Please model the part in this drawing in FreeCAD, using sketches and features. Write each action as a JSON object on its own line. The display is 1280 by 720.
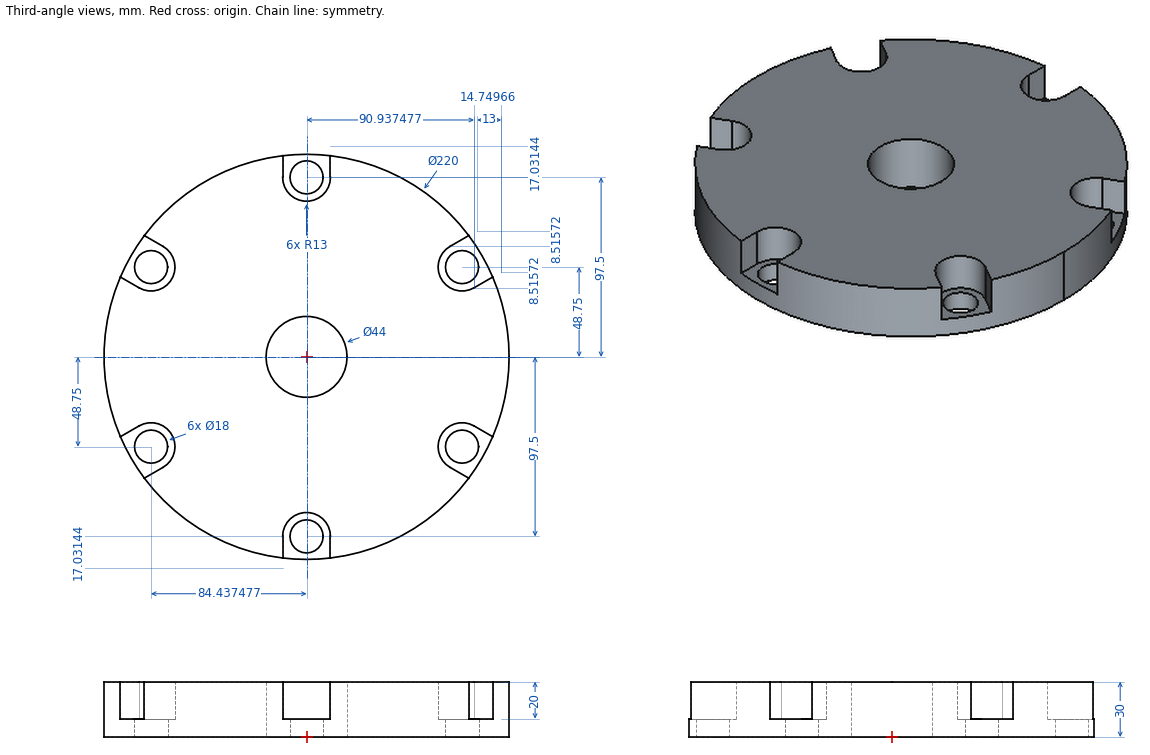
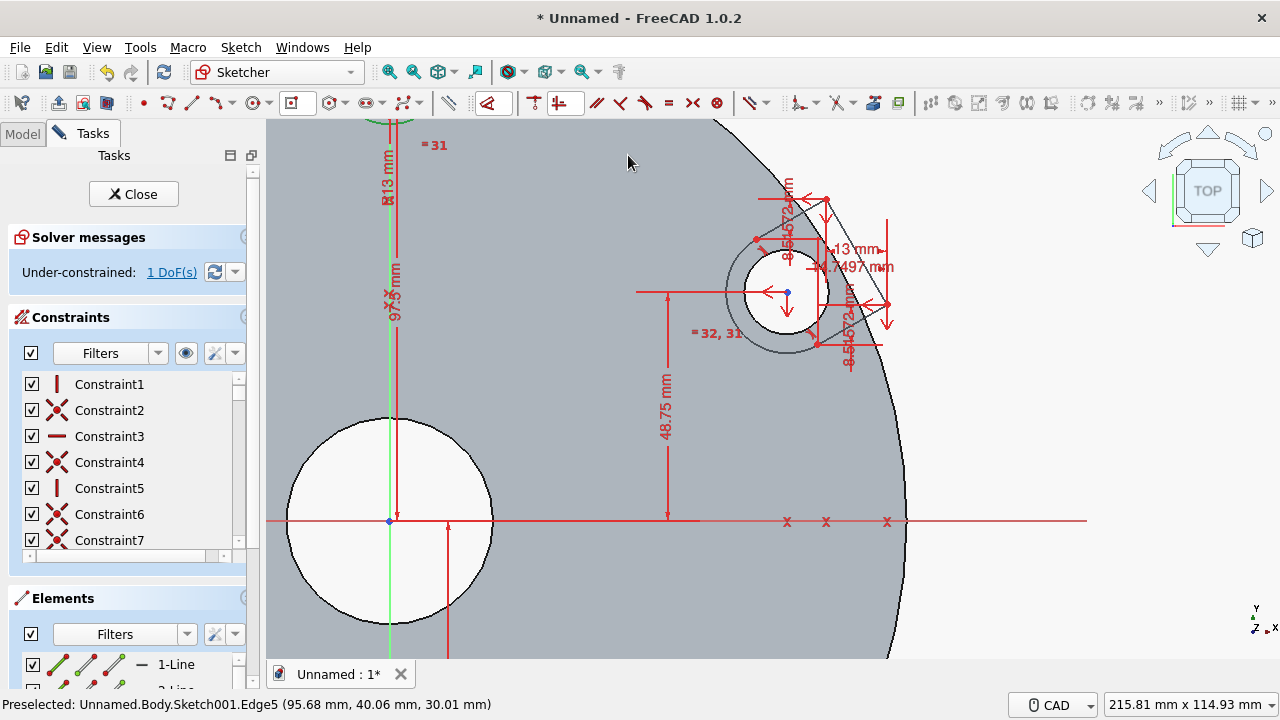
{"action": "left_click", "coordinate": [818, 345]}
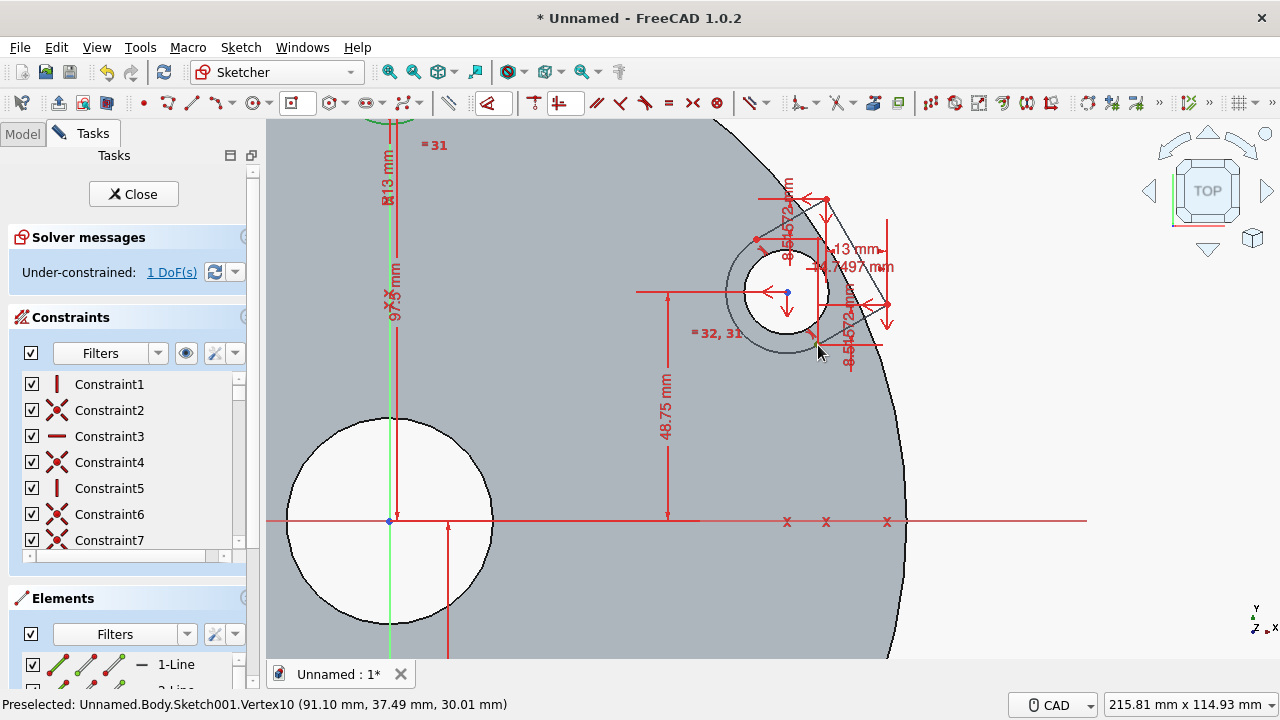
{"action": "left_click", "coordinate": [506, 104]}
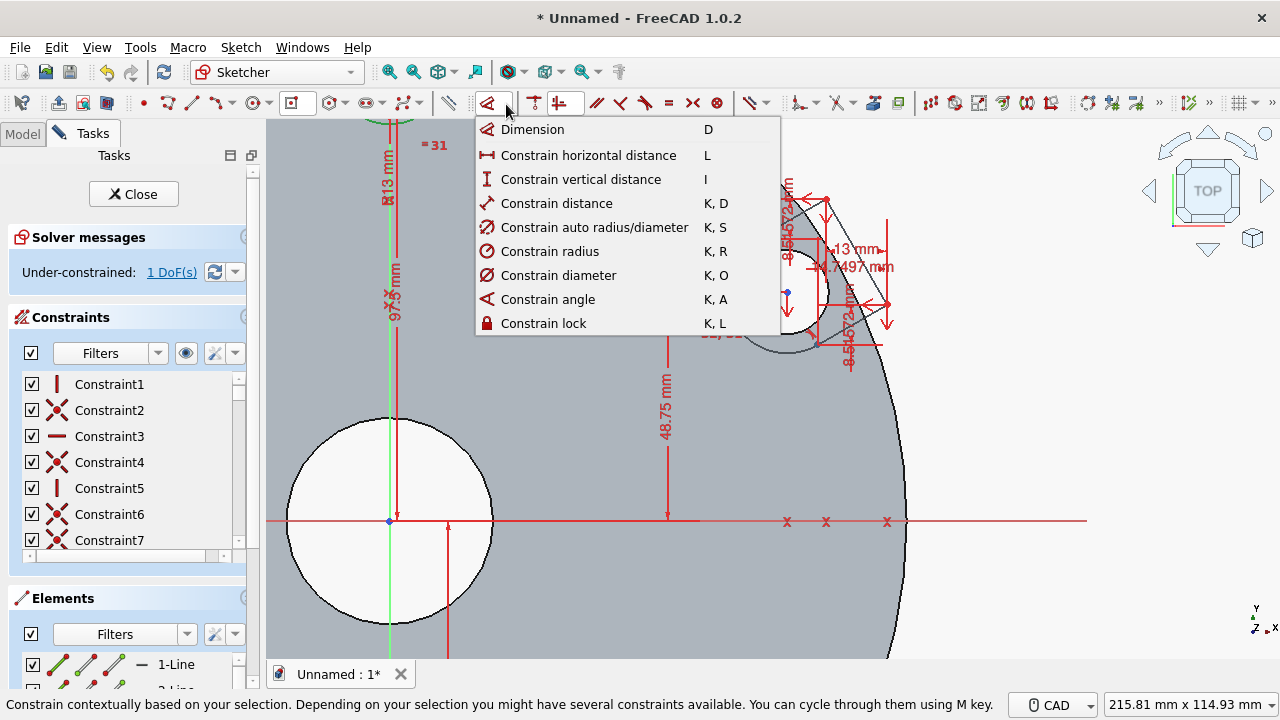
{"action": "left_click", "coordinate": [628, 155]}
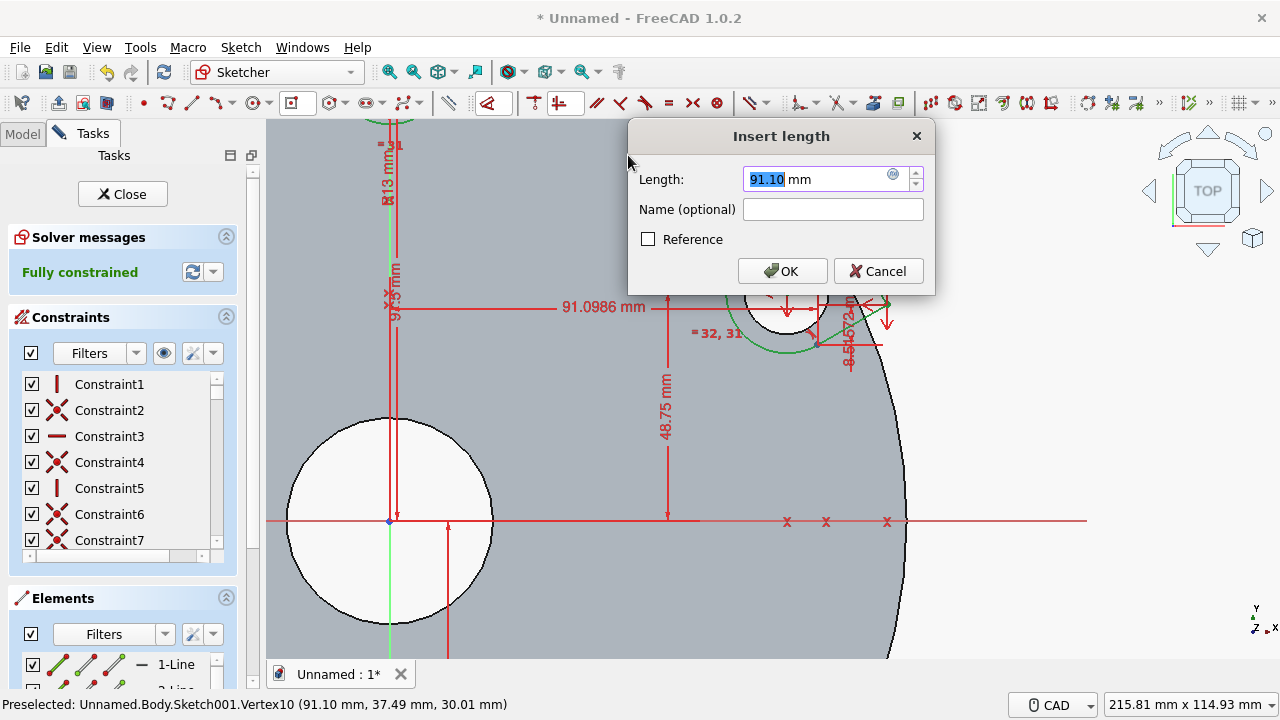
{"action": "type", "text": "90.937477"}
{"action": "key", "text": "Return"}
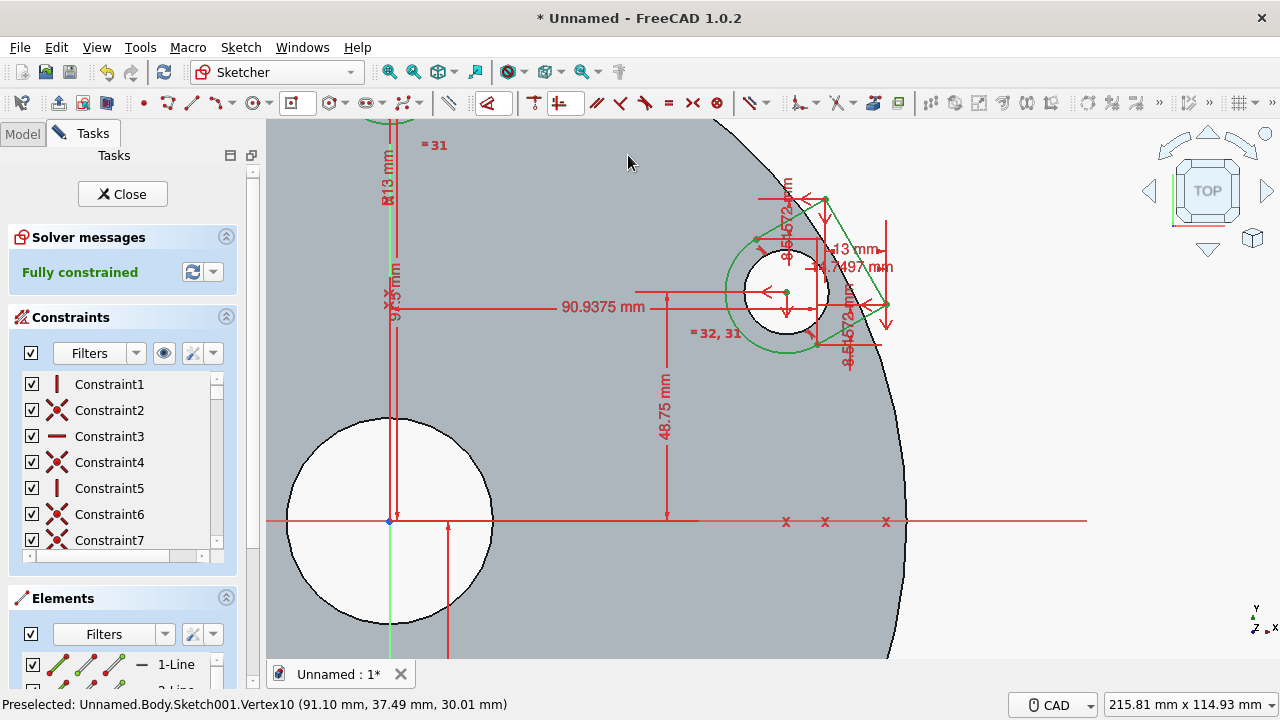
{"action": "left_click", "coordinate": [123, 194]}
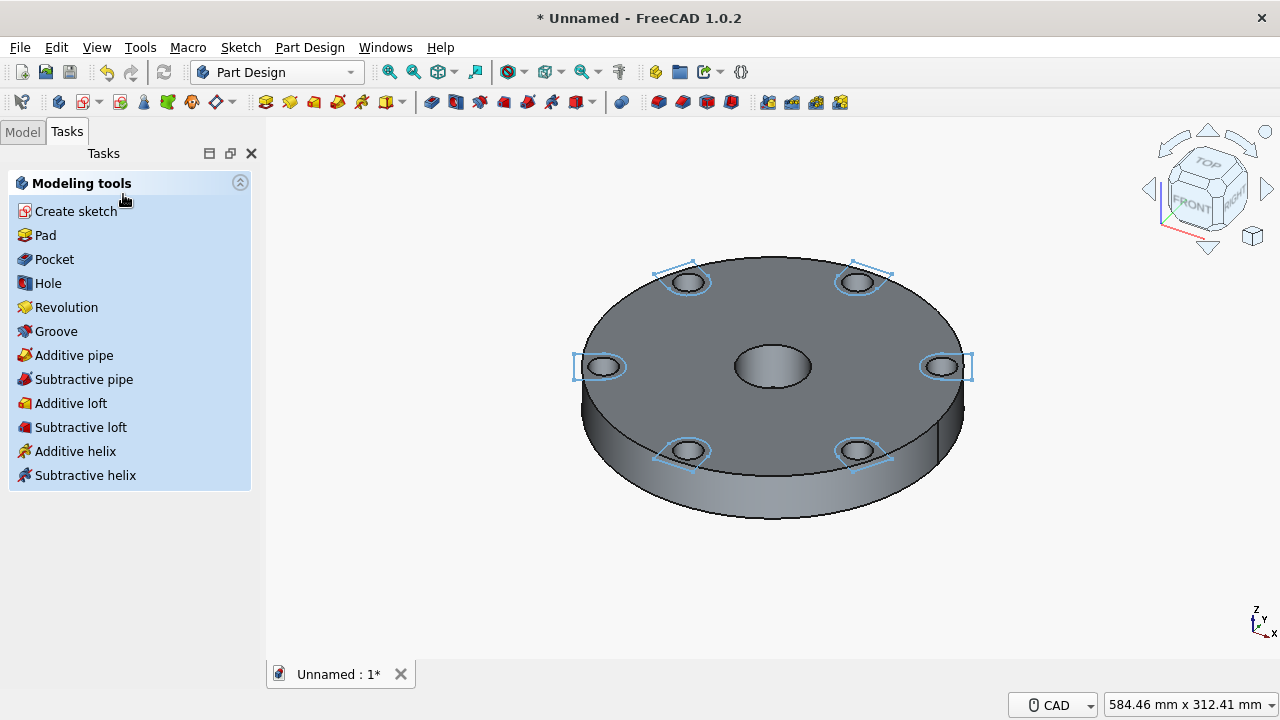
{"action": "left_click", "coordinate": [432, 102]}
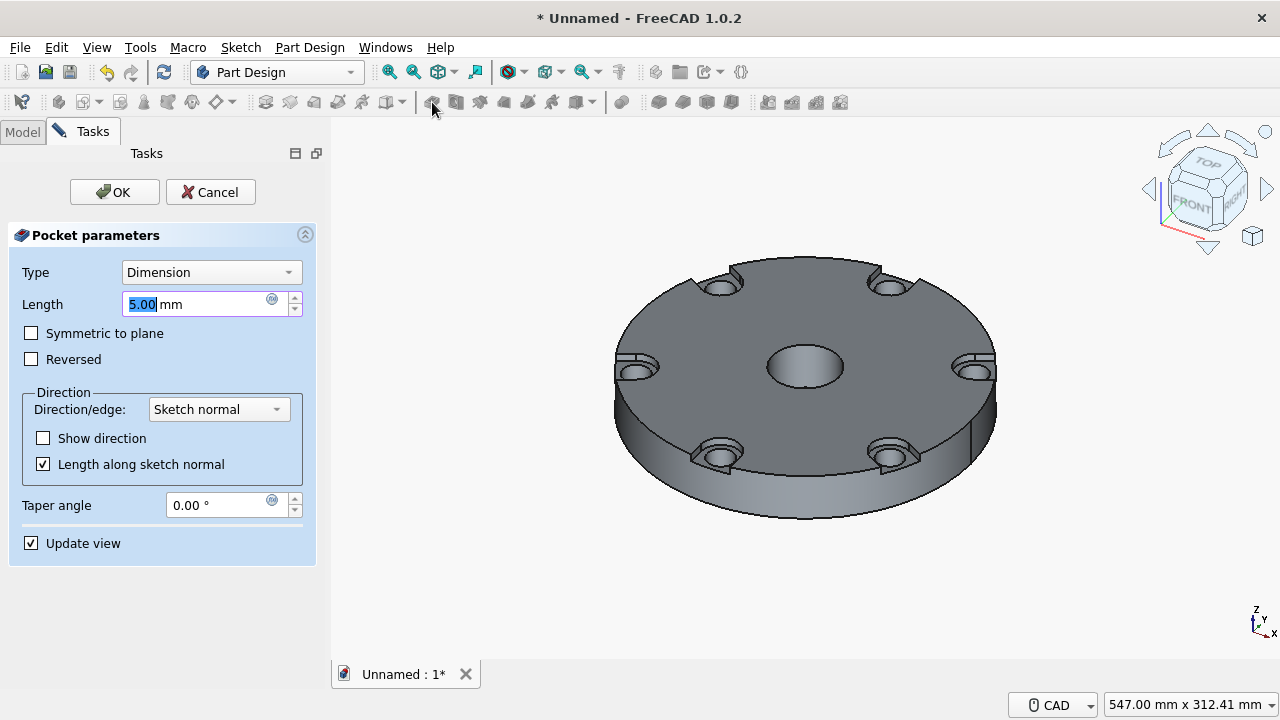
{"action": "type", "text": "20"}
{"action": "key", "text": "Tab"}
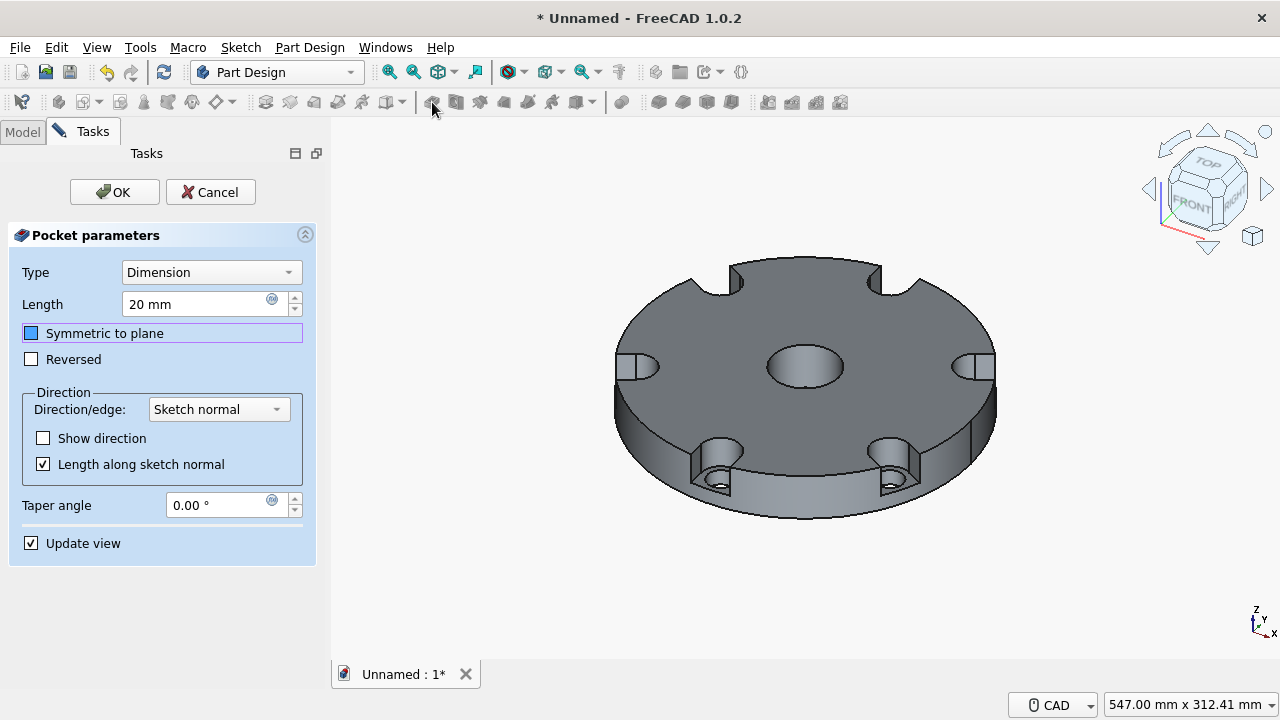
{"action": "left_click", "coordinate": [115, 192]}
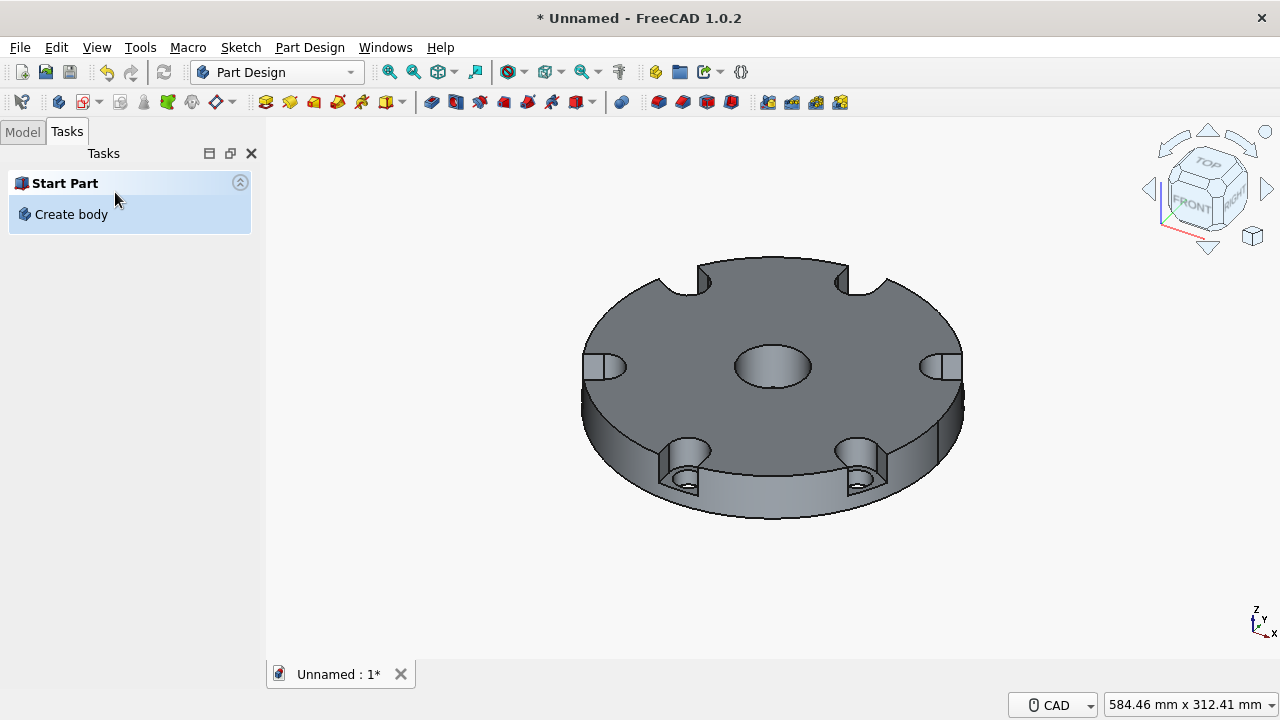
{"action": "key", "text": "0"}